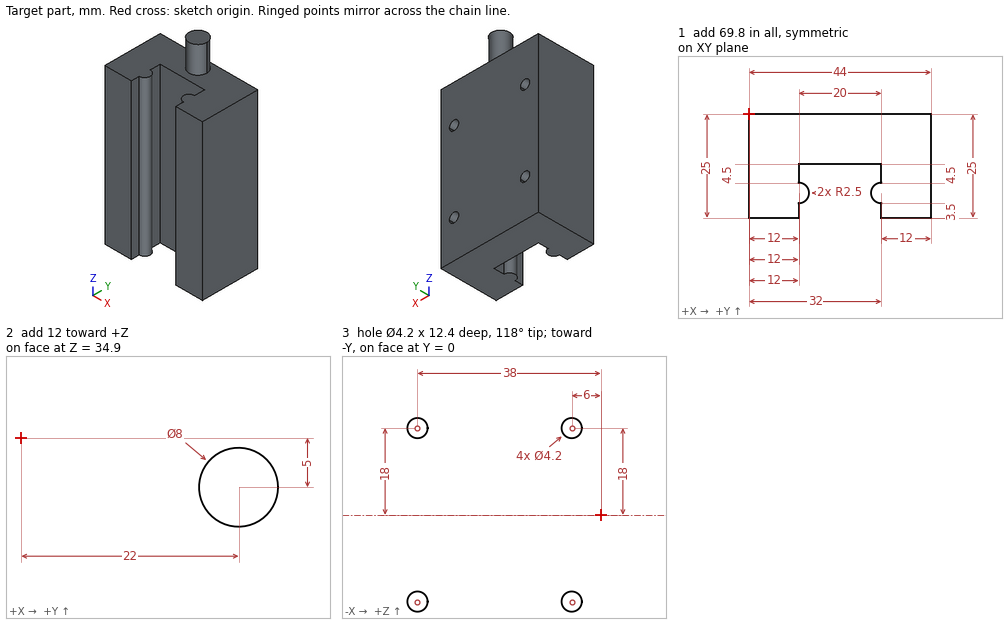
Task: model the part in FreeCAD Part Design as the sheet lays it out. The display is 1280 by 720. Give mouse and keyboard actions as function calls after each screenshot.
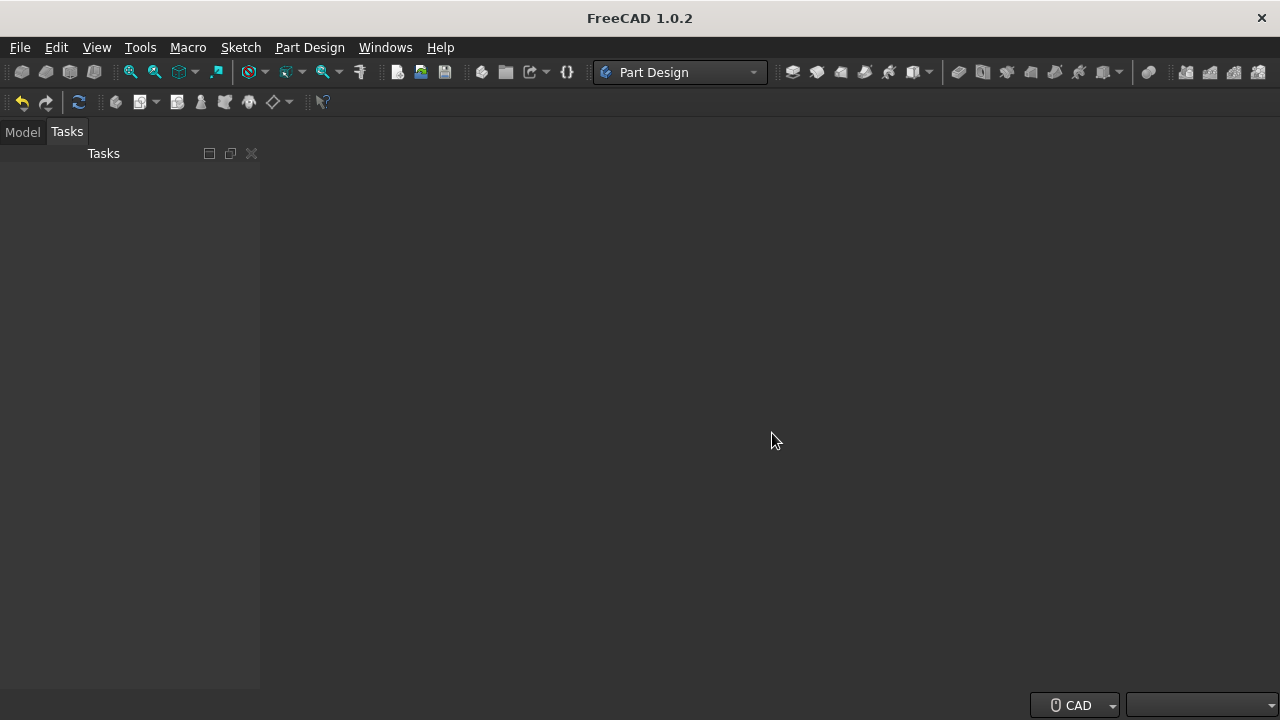
click(398, 72)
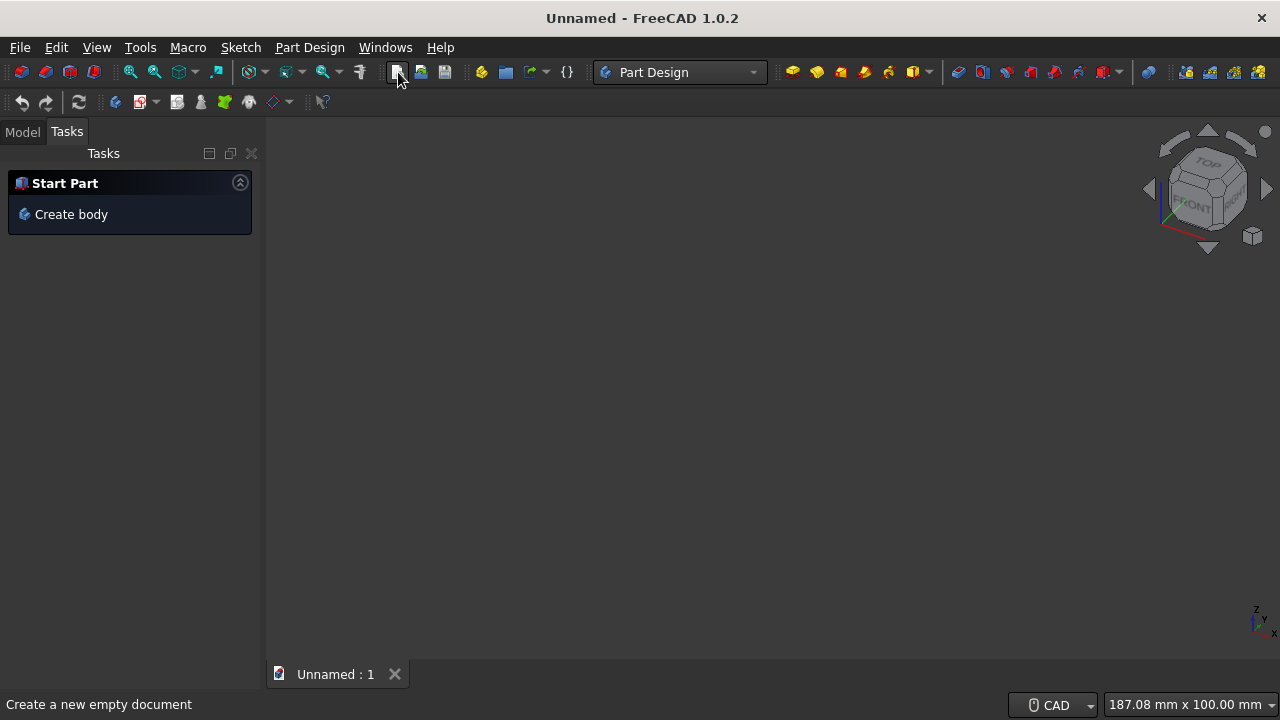
click(140, 102)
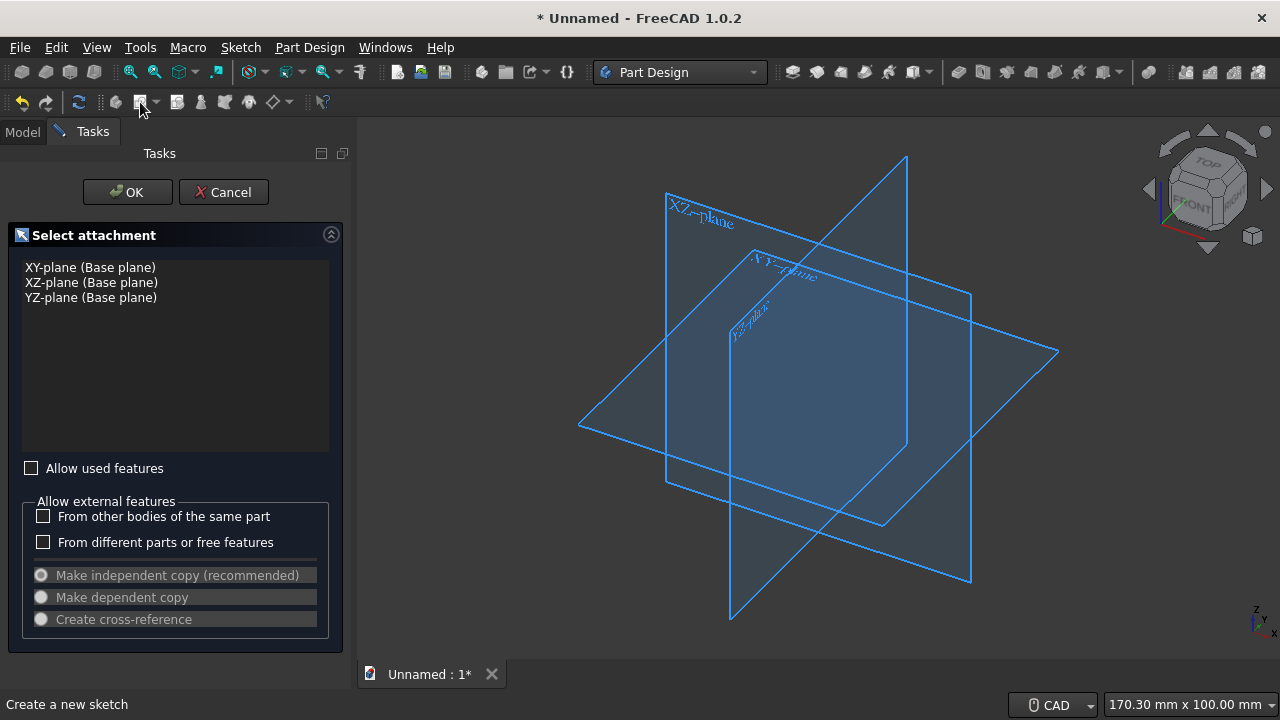
click(82, 268)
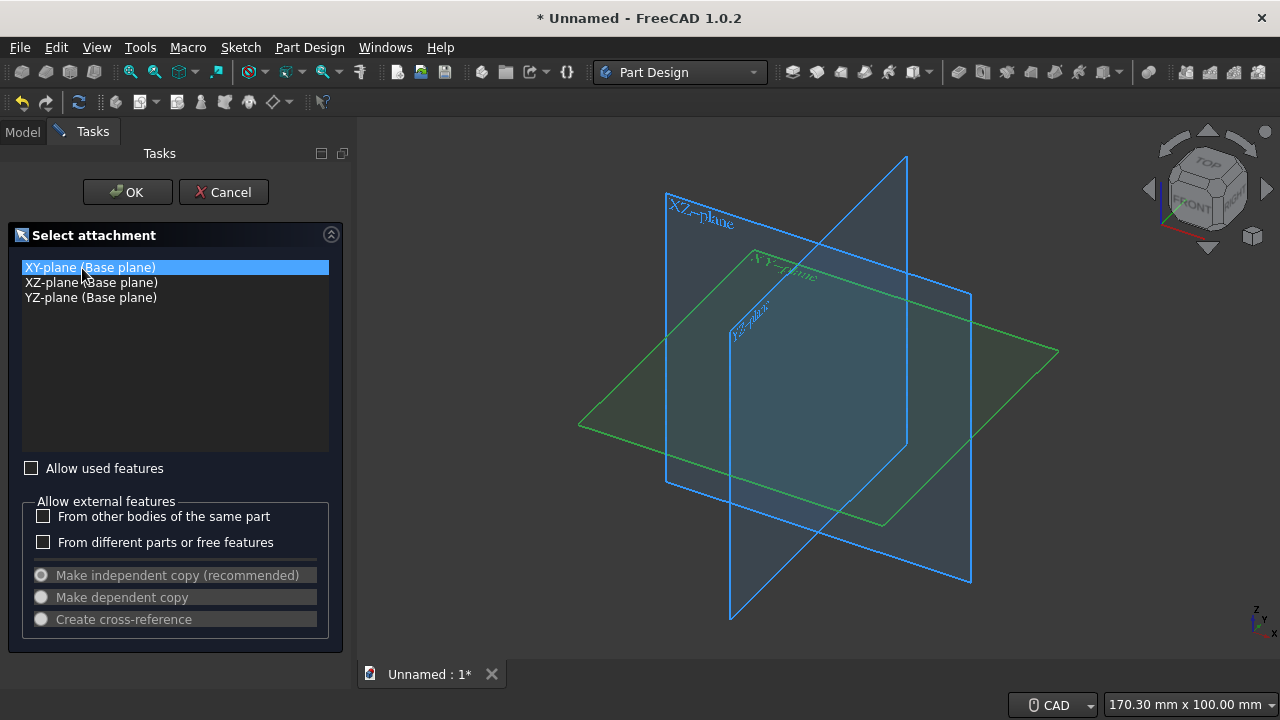
click(128, 192)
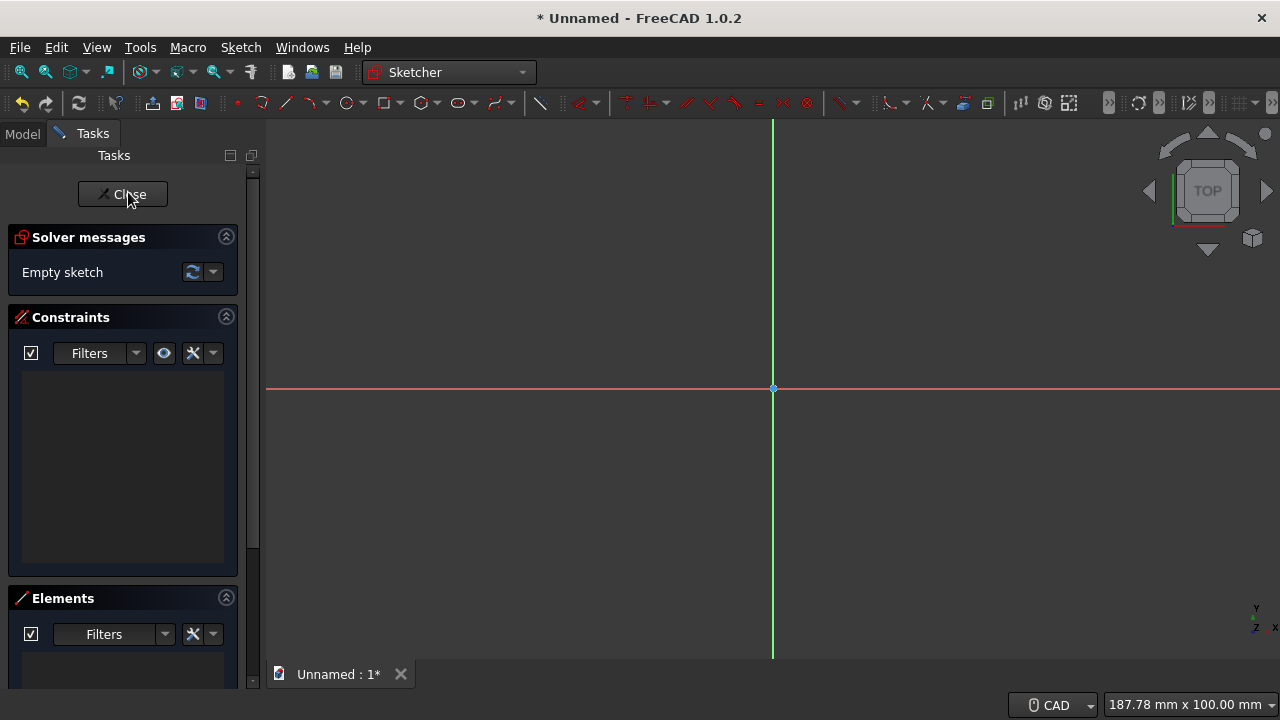
scroll(1045, 512, up, 4)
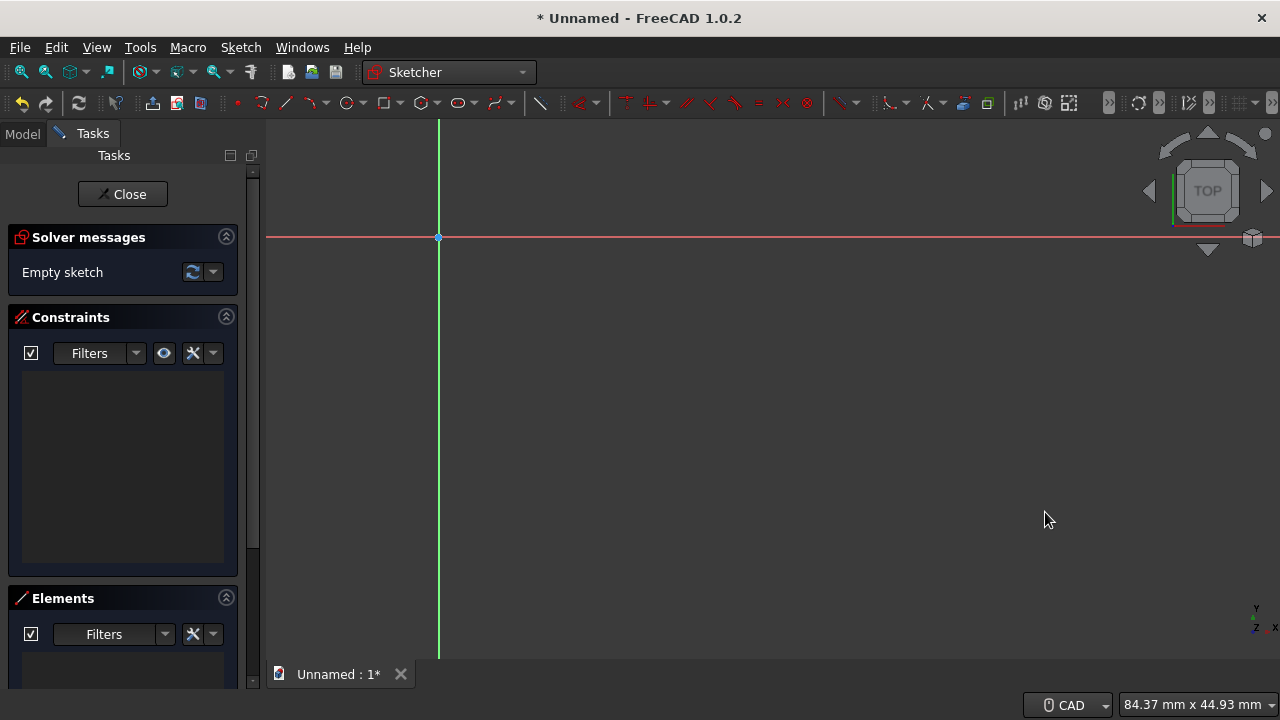
click(262, 104)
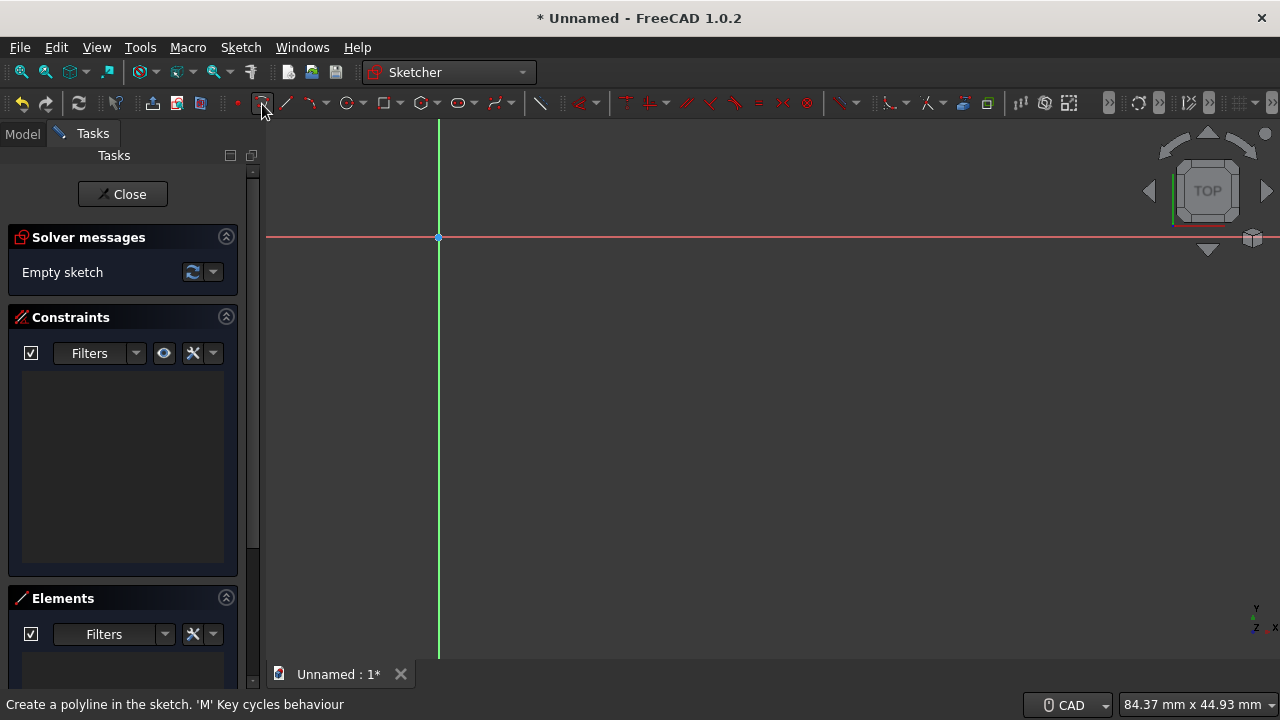
click(583, 436)
click(583, 382)
click(823, 382)
click(823, 436)
right_click(823, 436)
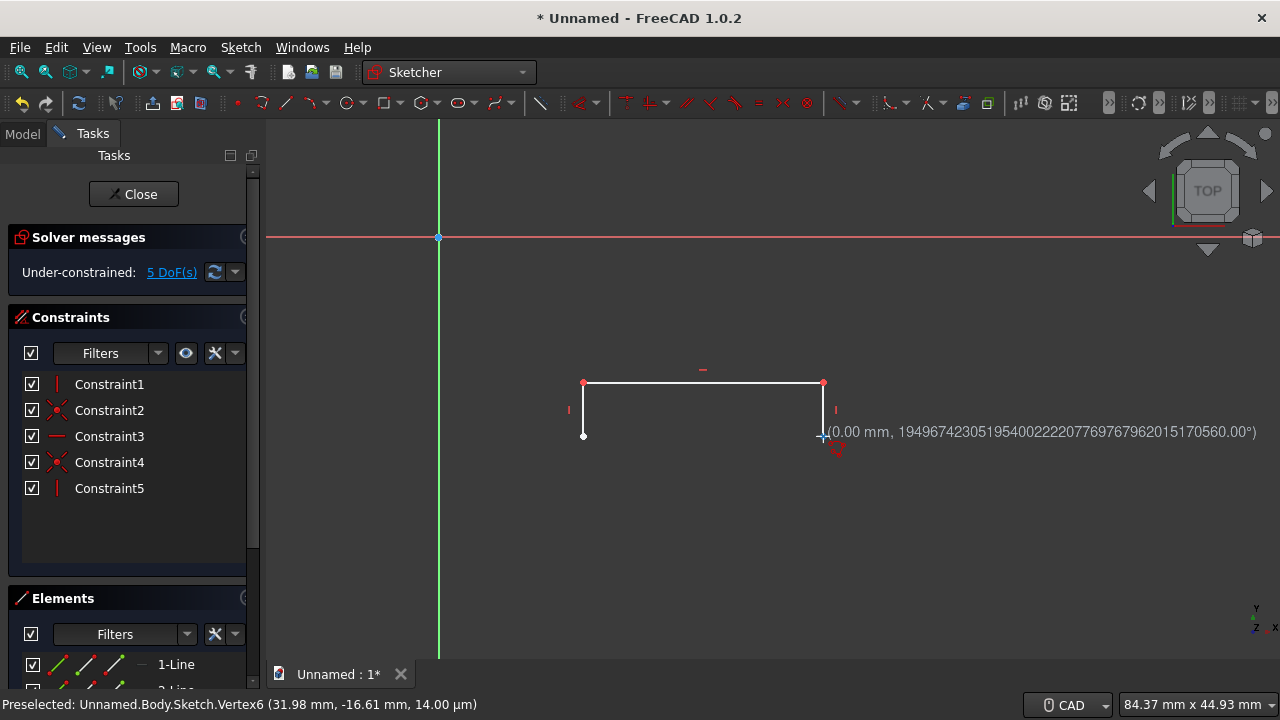
click(823, 496)
click(823, 538)
click(967, 538)
click(967, 237)
click(439, 237)
click(448, 538)
click(583, 538)
click(583, 496)
right_click(583, 496)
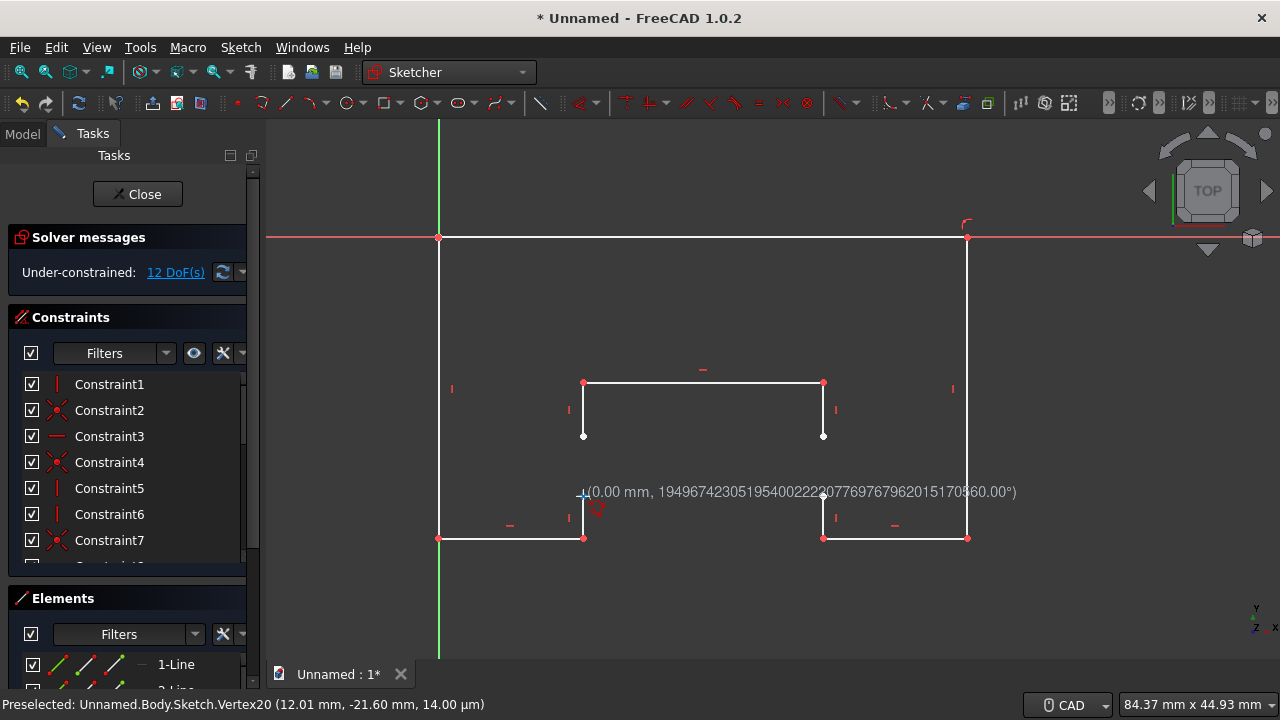
click(310, 104)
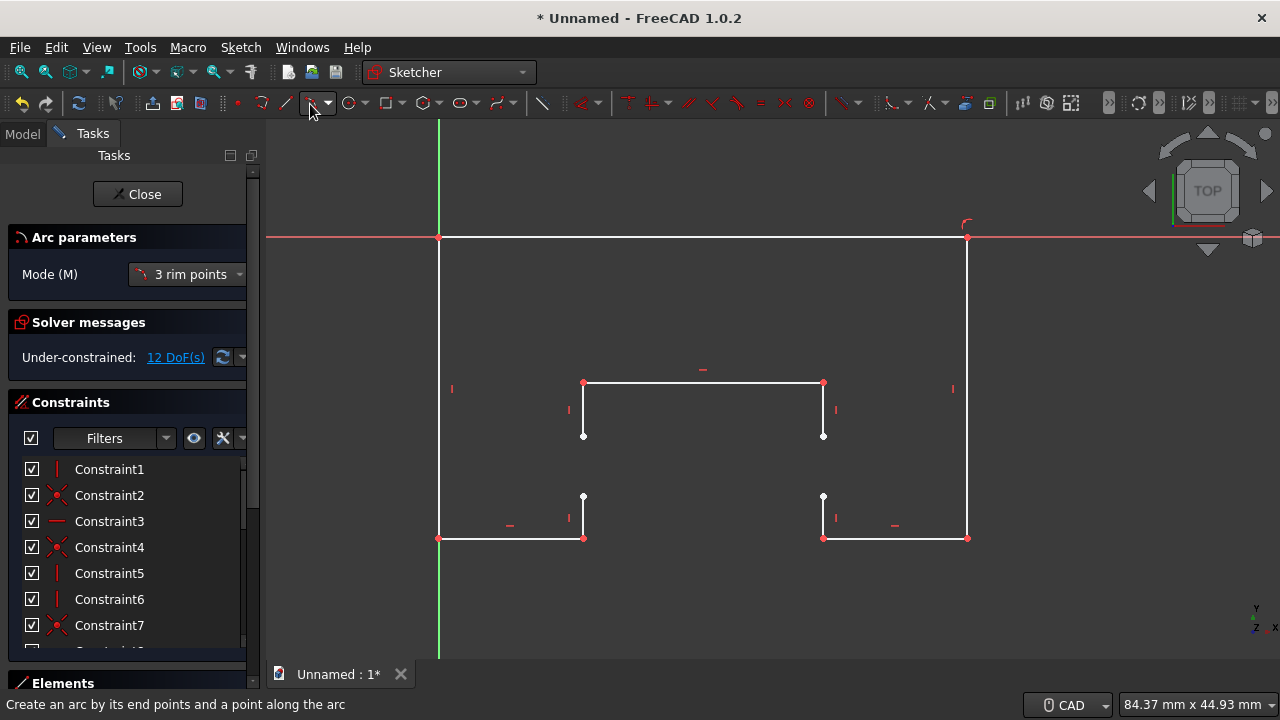
click(823, 437)
click(823, 497)
click(793, 466)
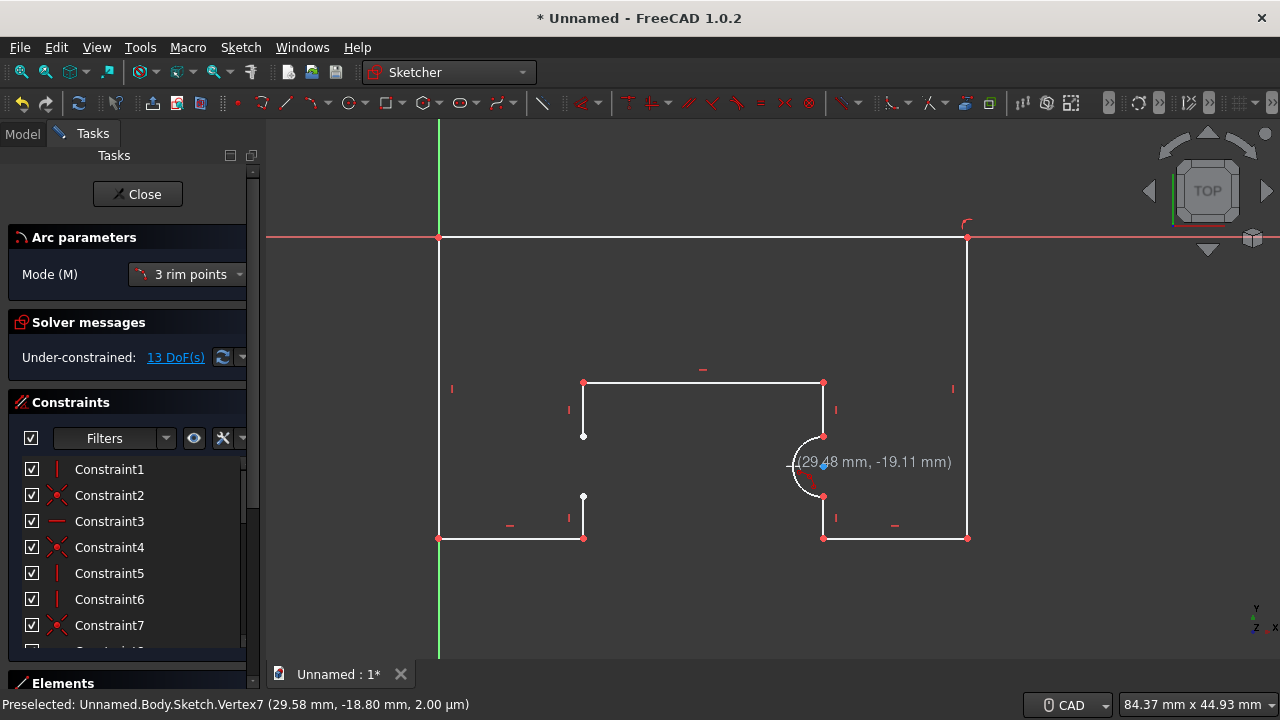
click(583, 497)
click(583, 437)
click(613, 466)
key(Escape)